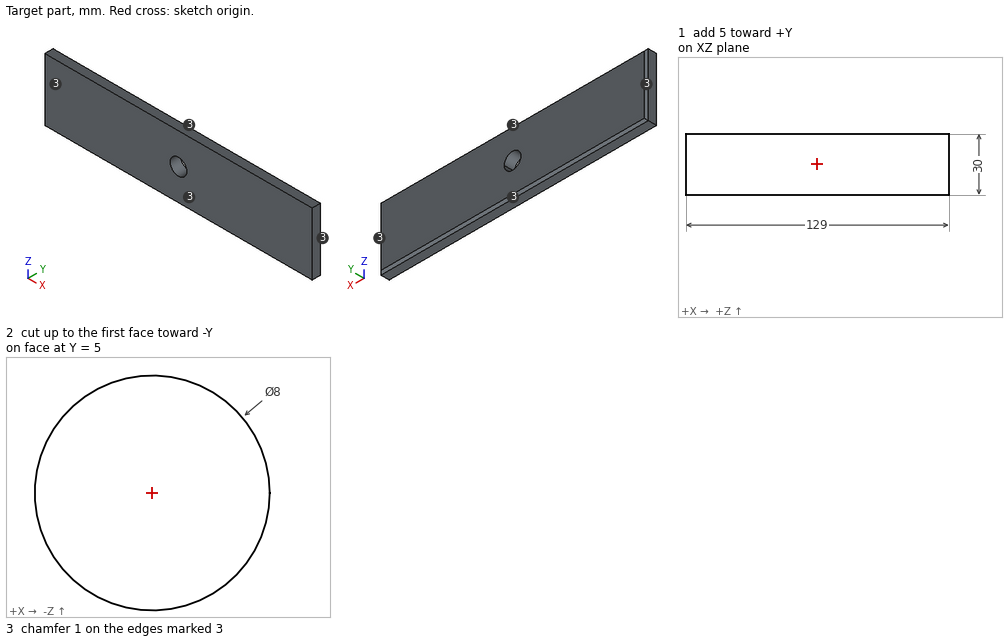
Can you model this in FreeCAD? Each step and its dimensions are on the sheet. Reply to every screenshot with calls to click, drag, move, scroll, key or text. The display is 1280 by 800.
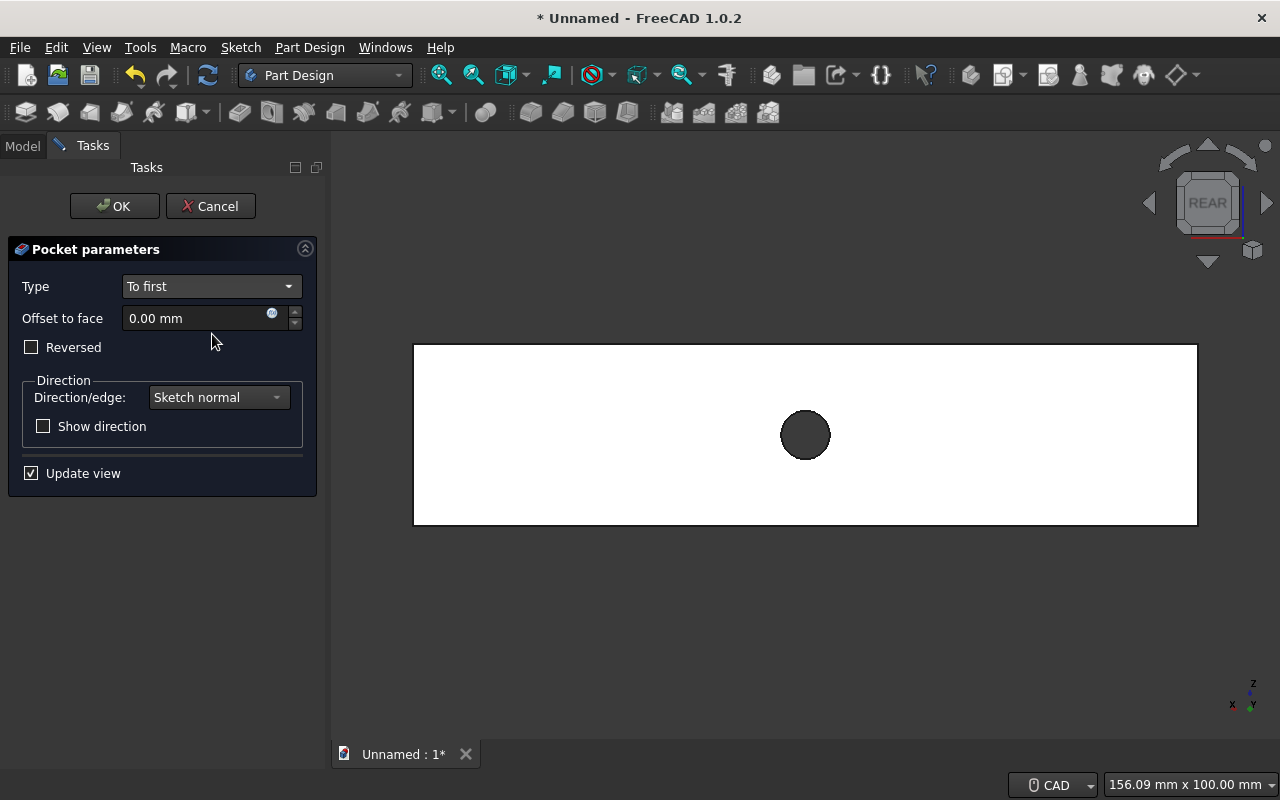
click(115, 206)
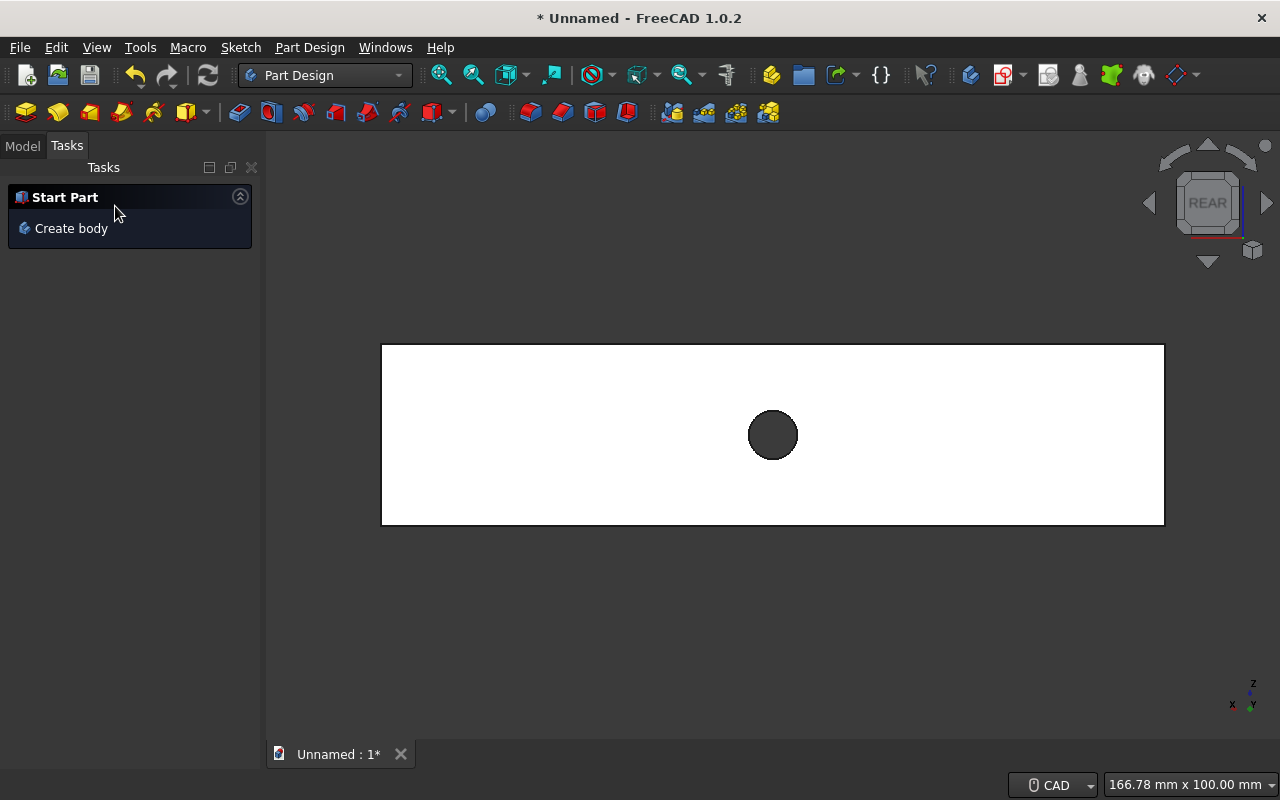
click(1165, 434)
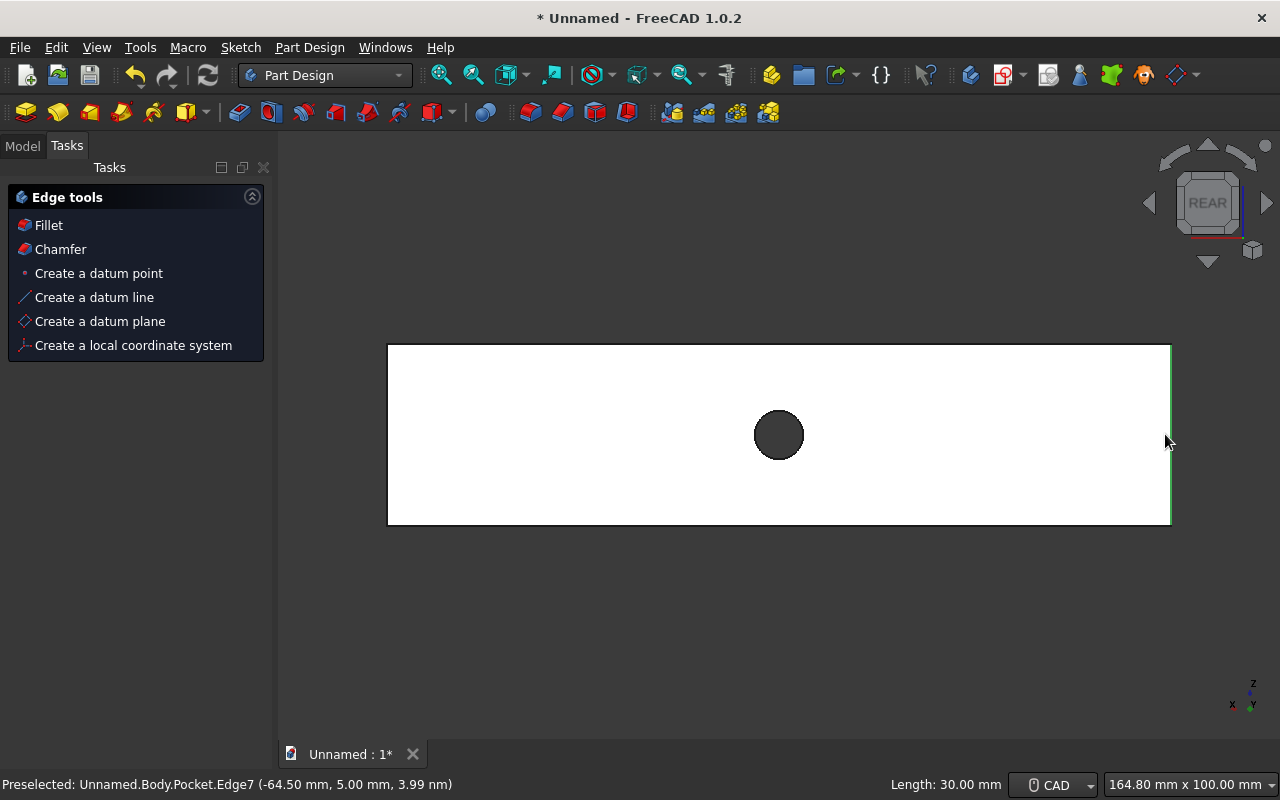
click(779, 525, ctrl)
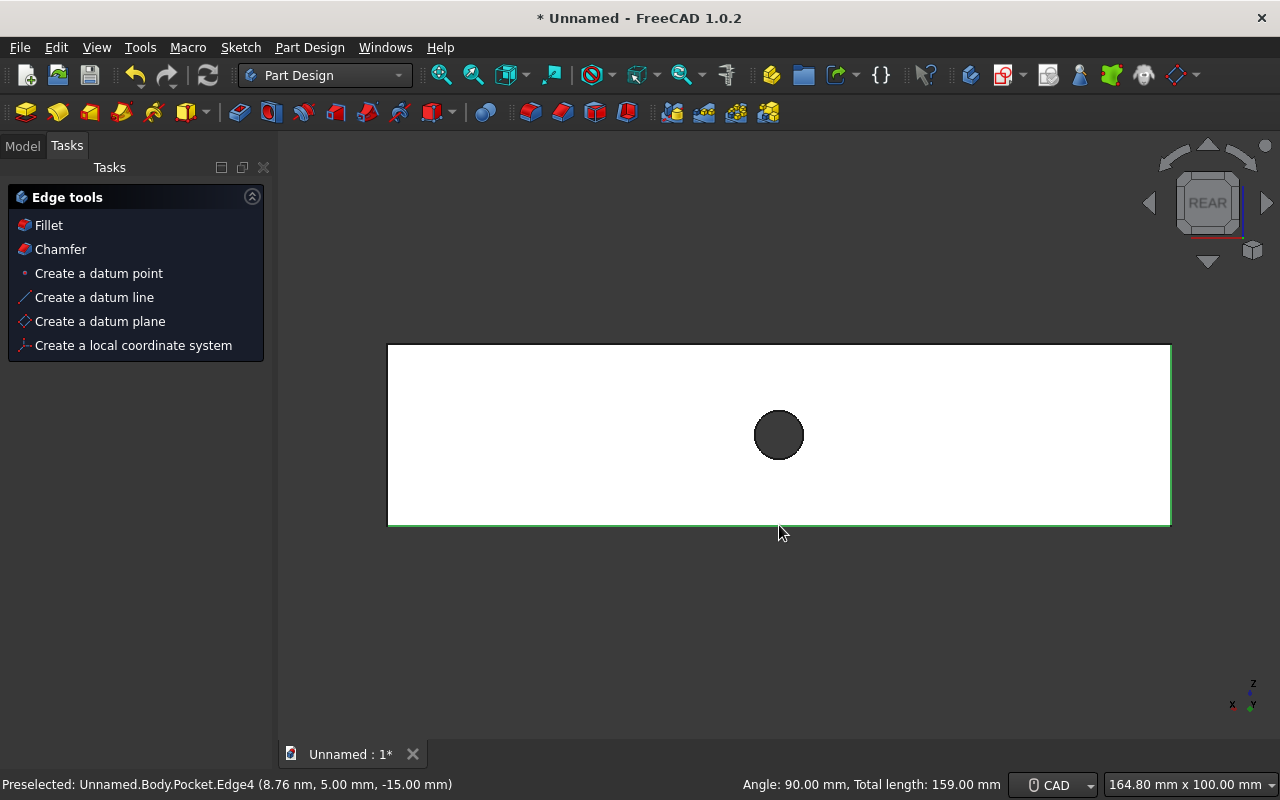
key(0)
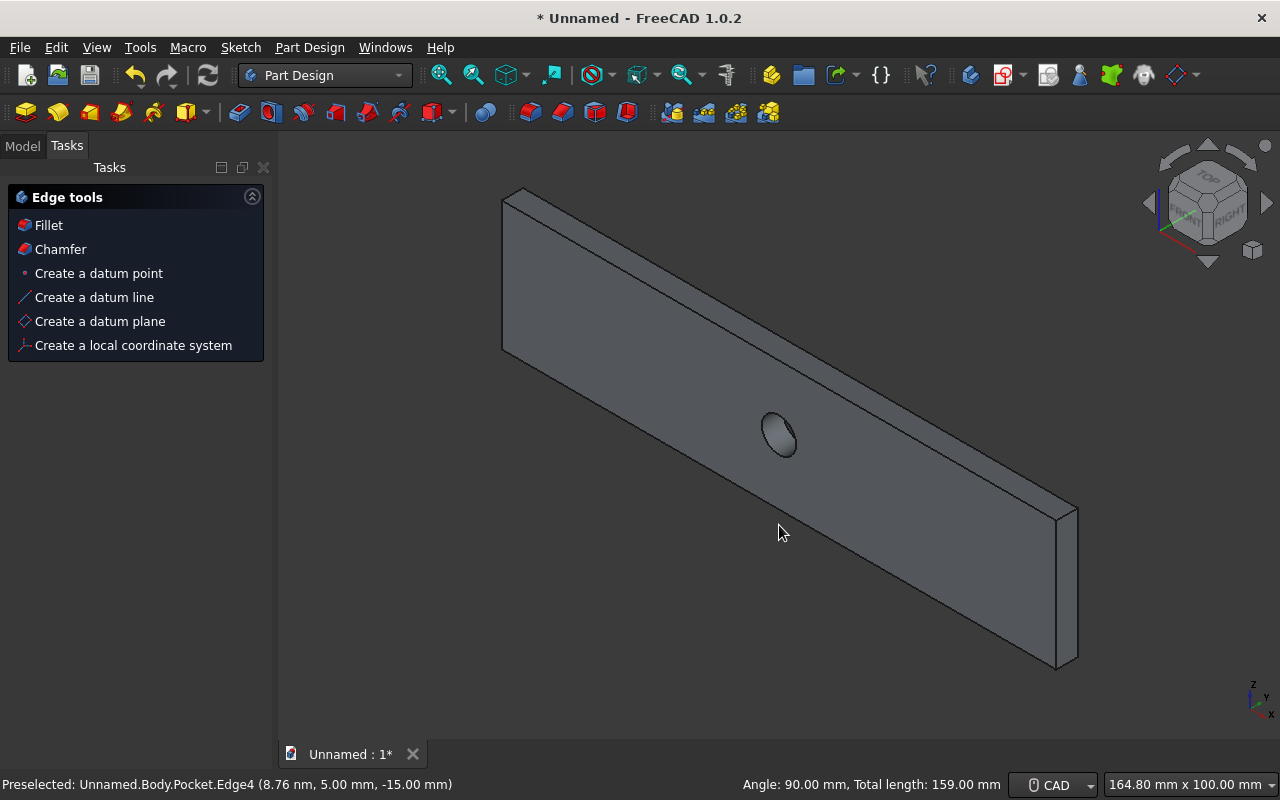
key(2)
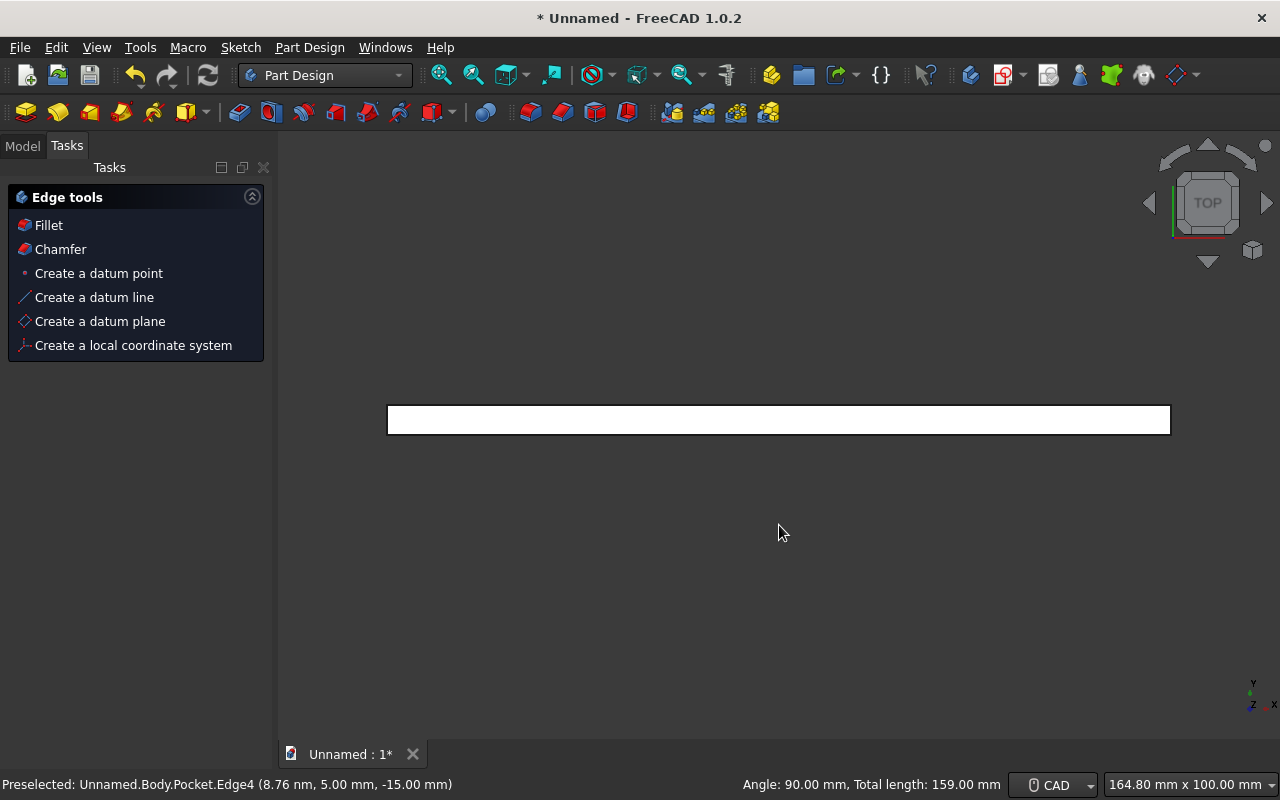
click(779, 404, ctrl)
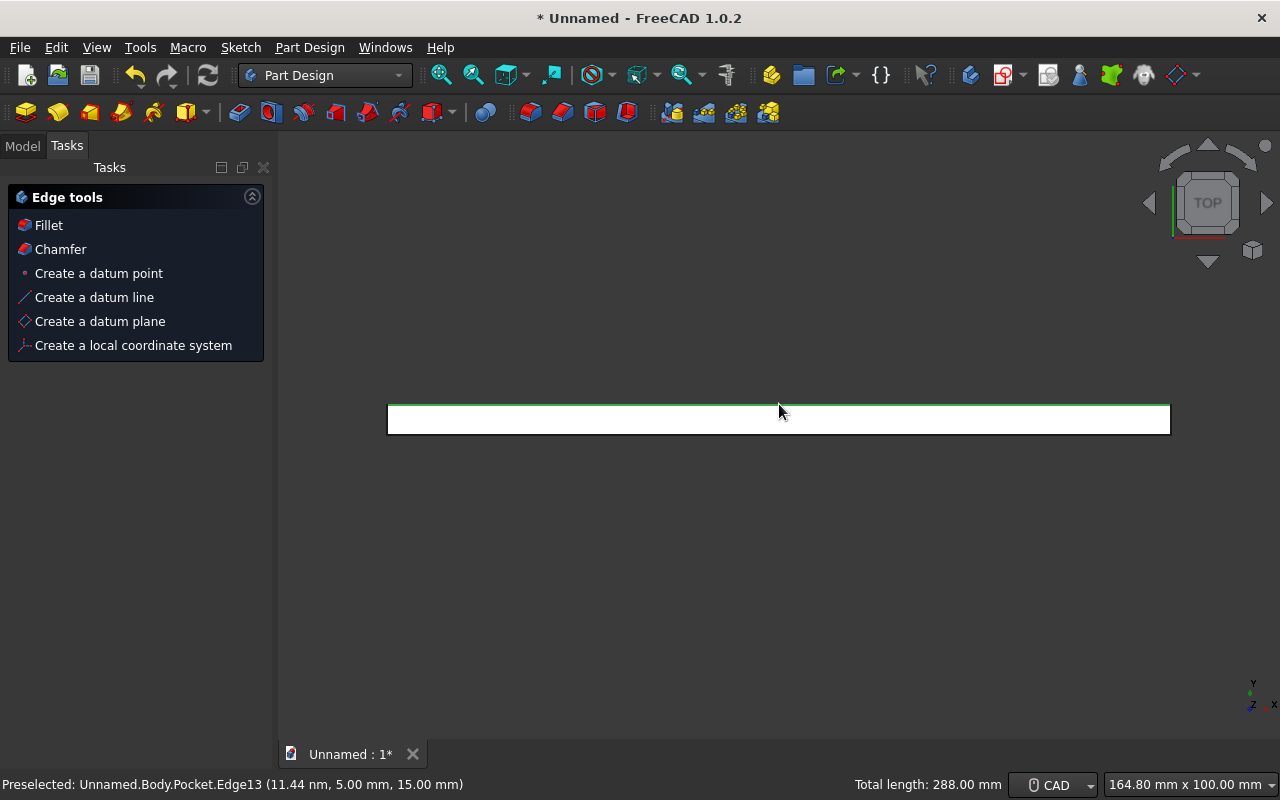
key(1)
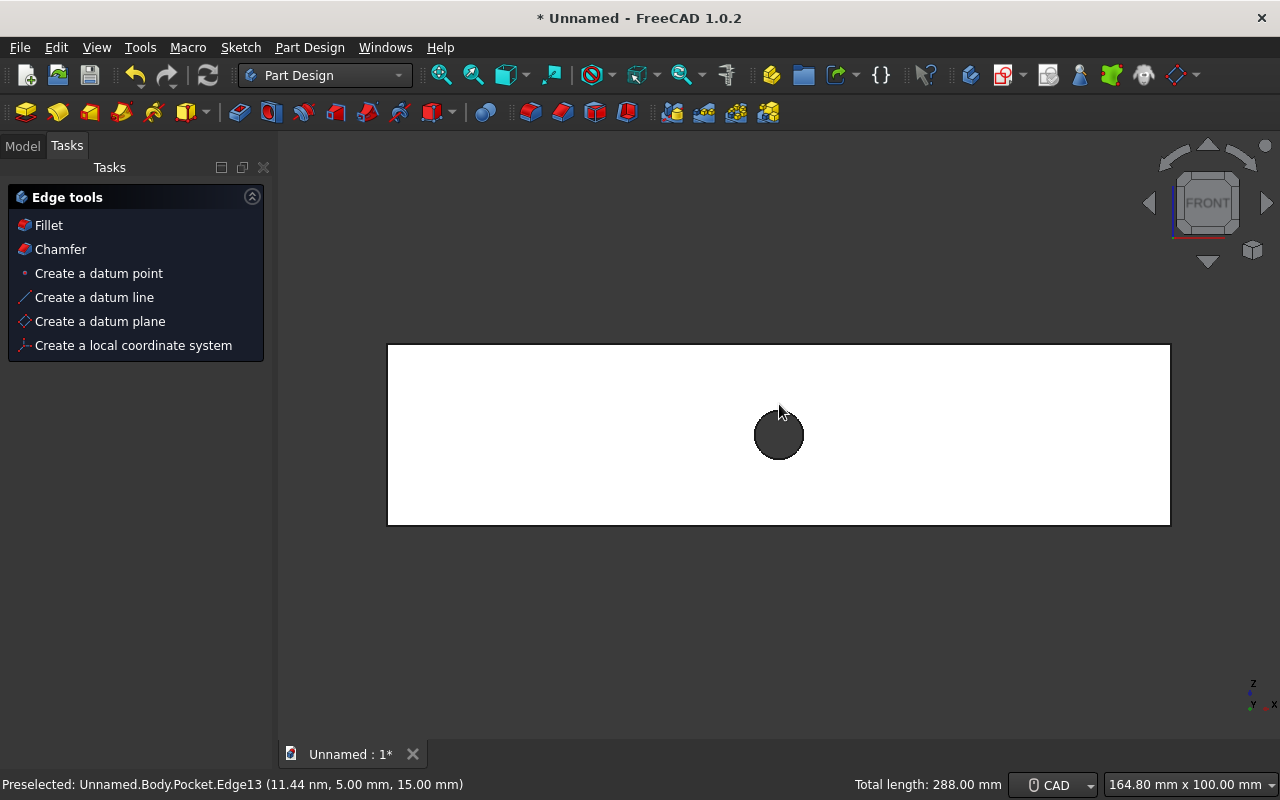
key(3)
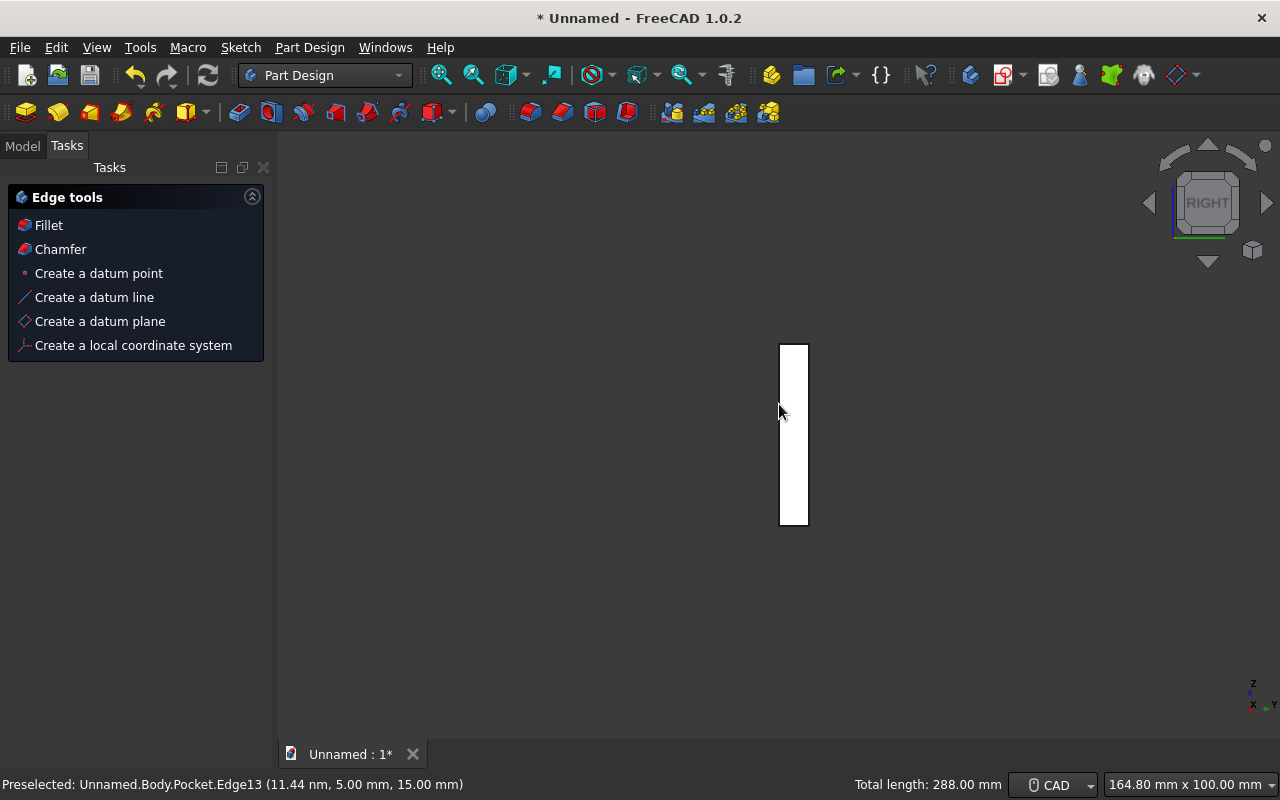
key(v)
key(f)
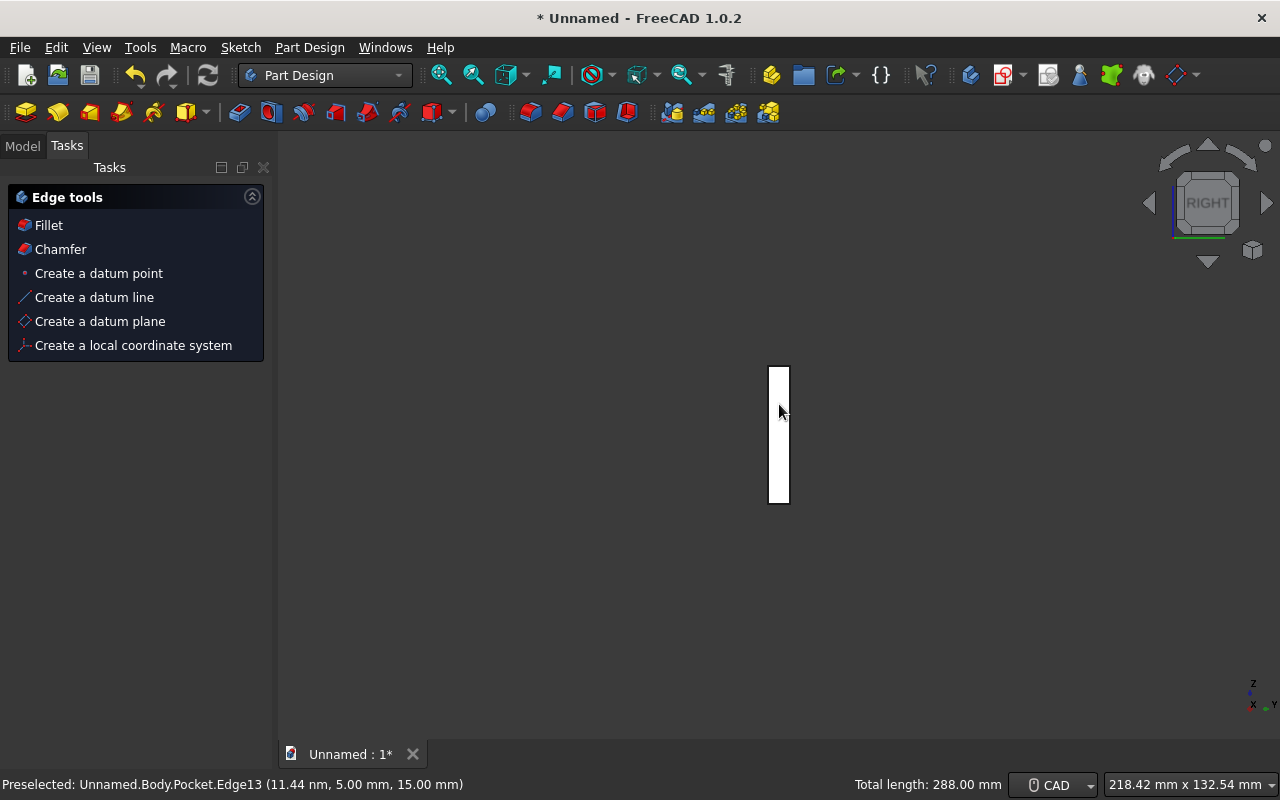
click(790, 434, ctrl)